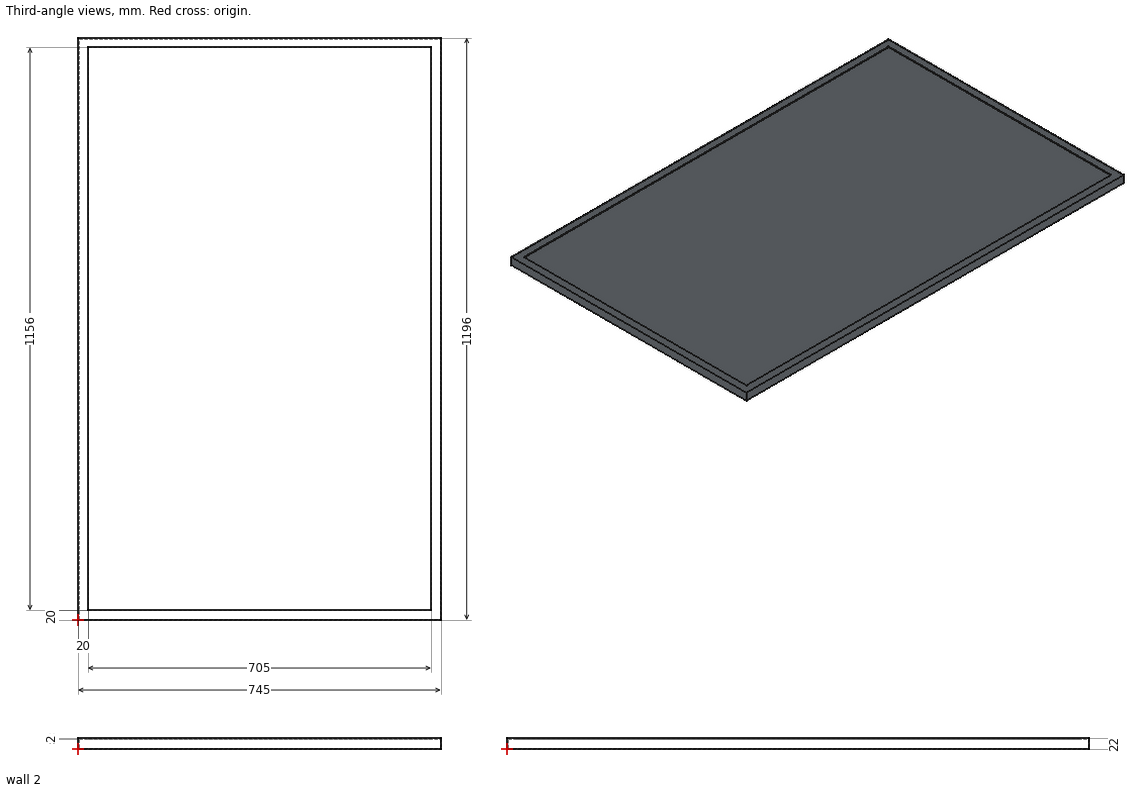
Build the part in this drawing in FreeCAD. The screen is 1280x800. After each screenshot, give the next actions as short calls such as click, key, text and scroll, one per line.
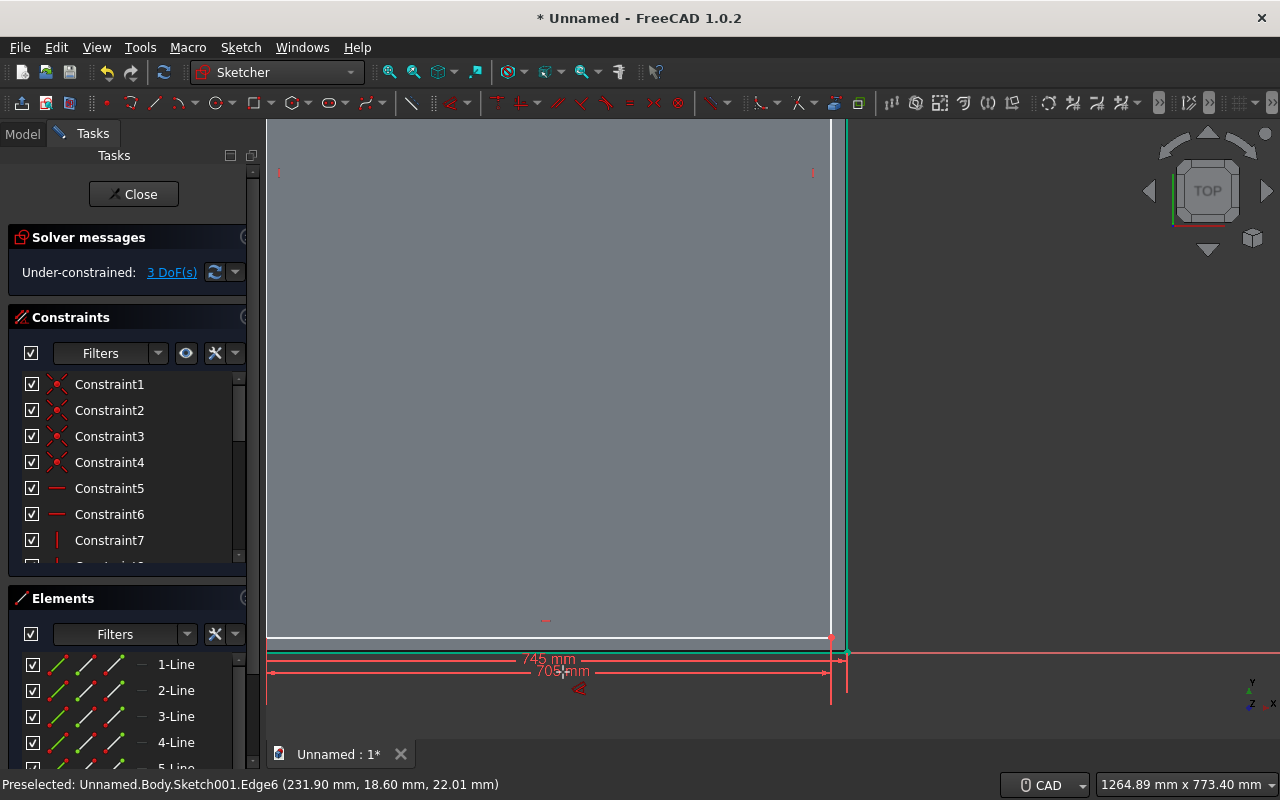
scroll(832, 637, down, 4)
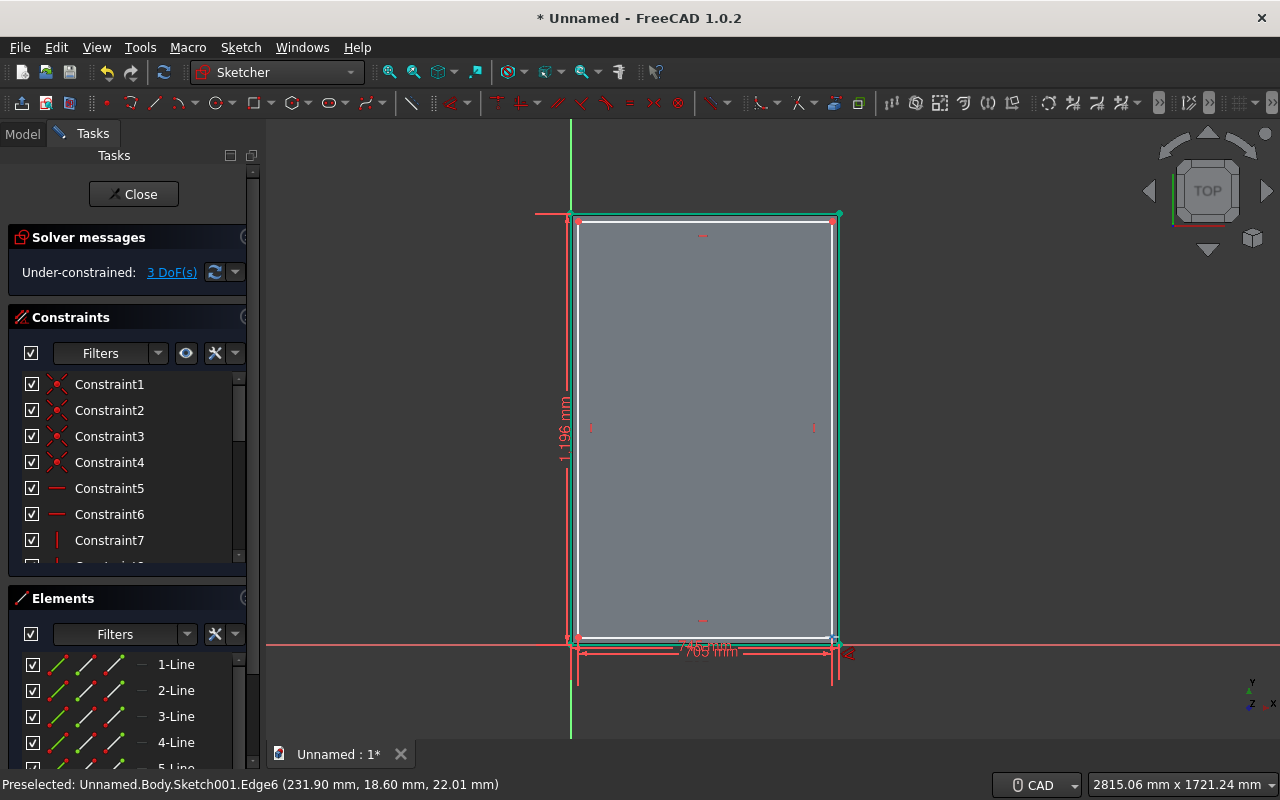
scroll(578, 222, up, 9)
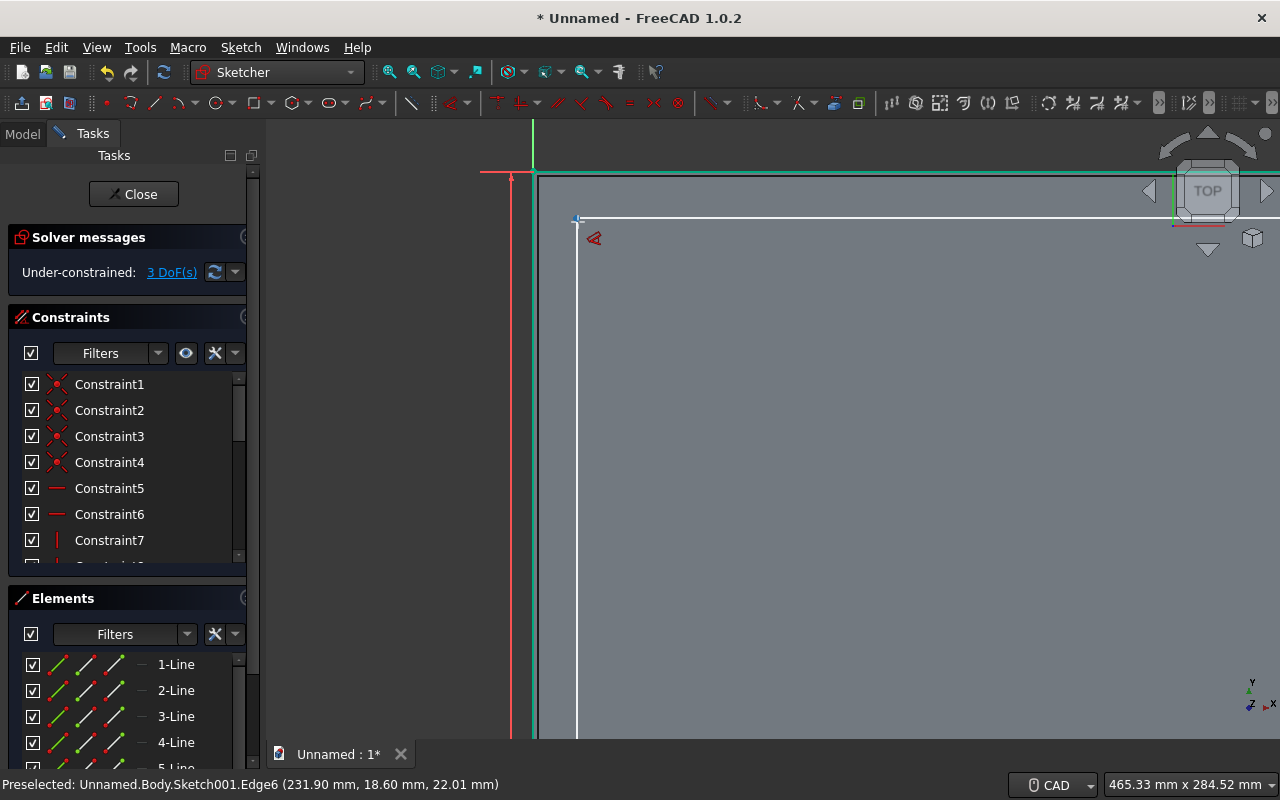
click(577, 218)
click(555, 184)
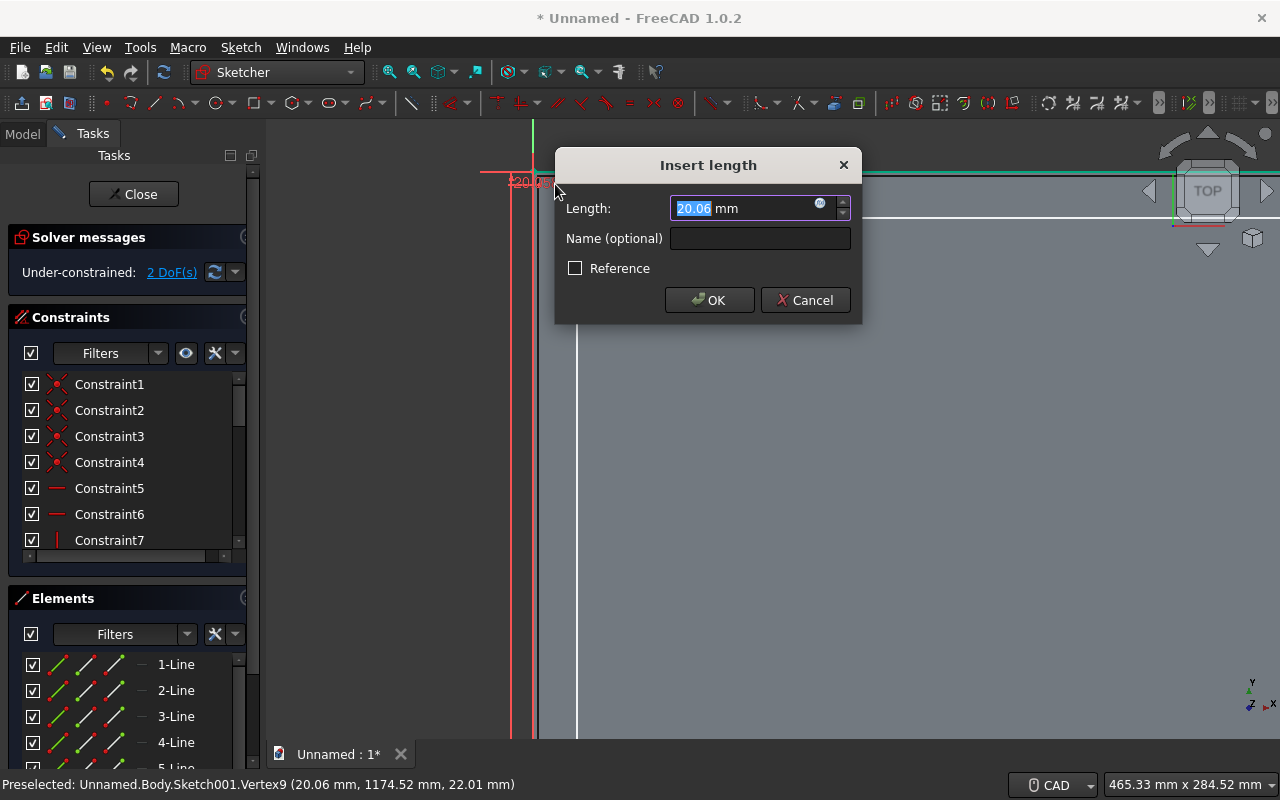
text(20)
key(Return)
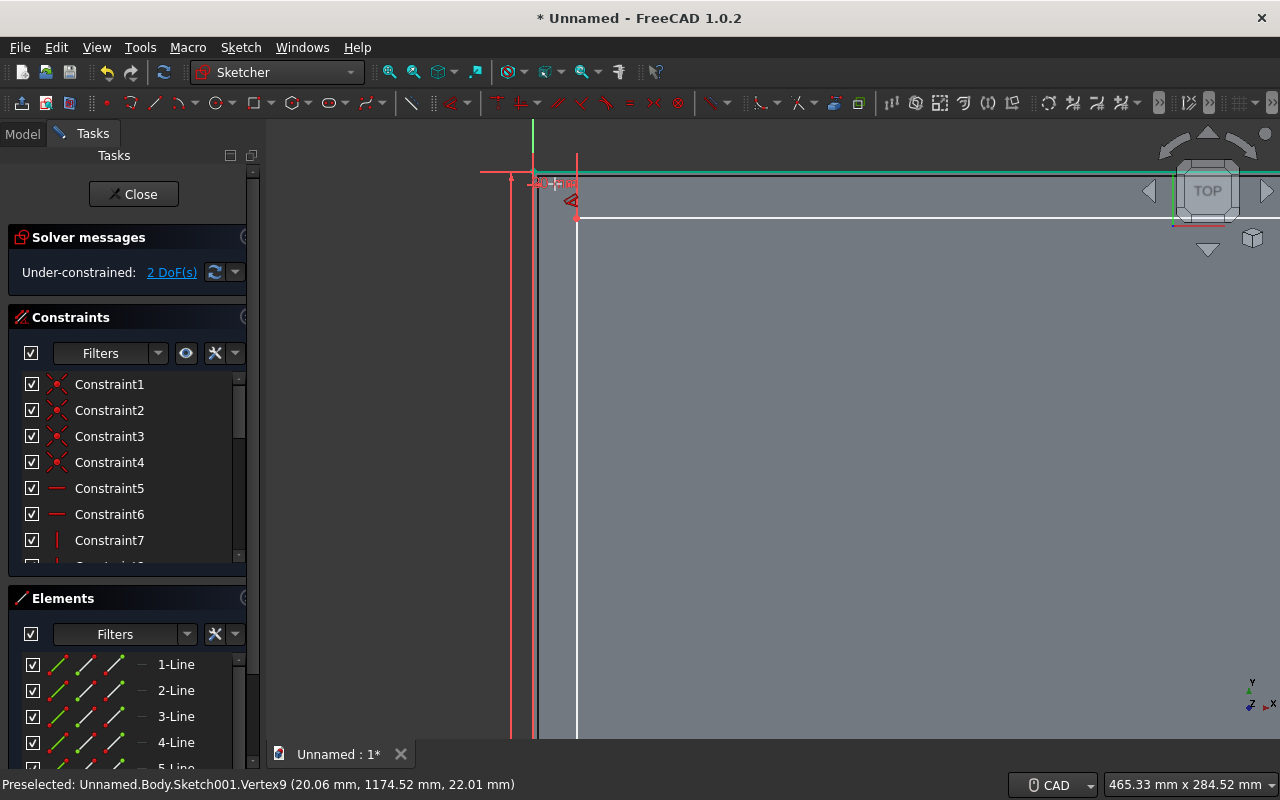
scroll(578, 222, down, 9)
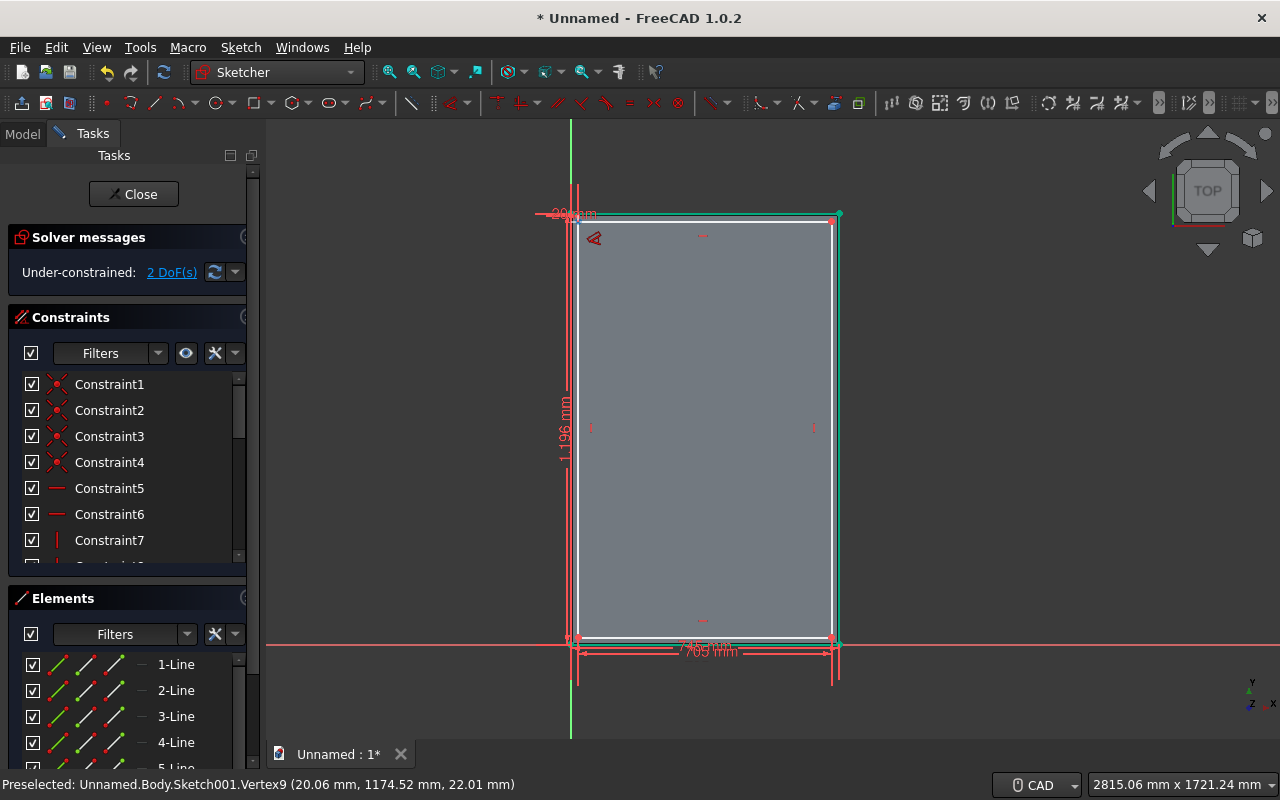
scroll(578, 638, up, 9)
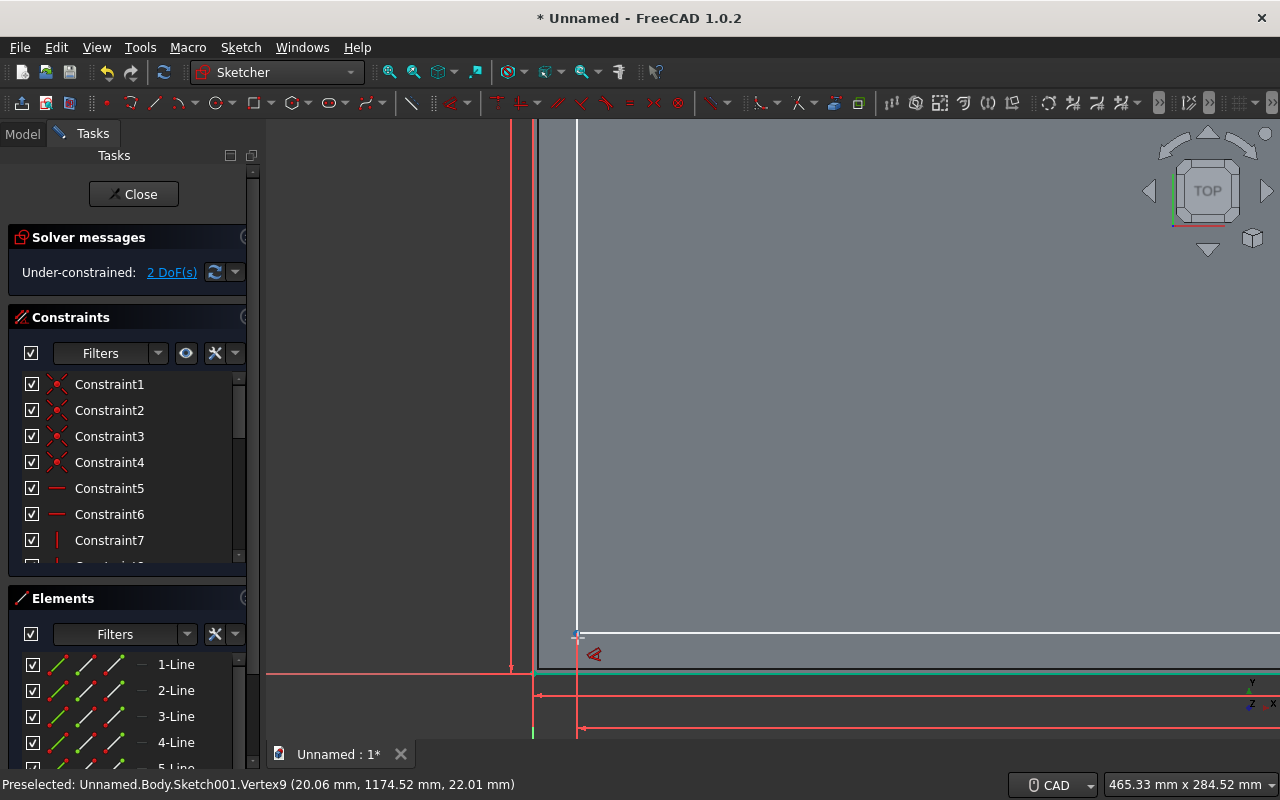
click(577, 633)
click(499, 653)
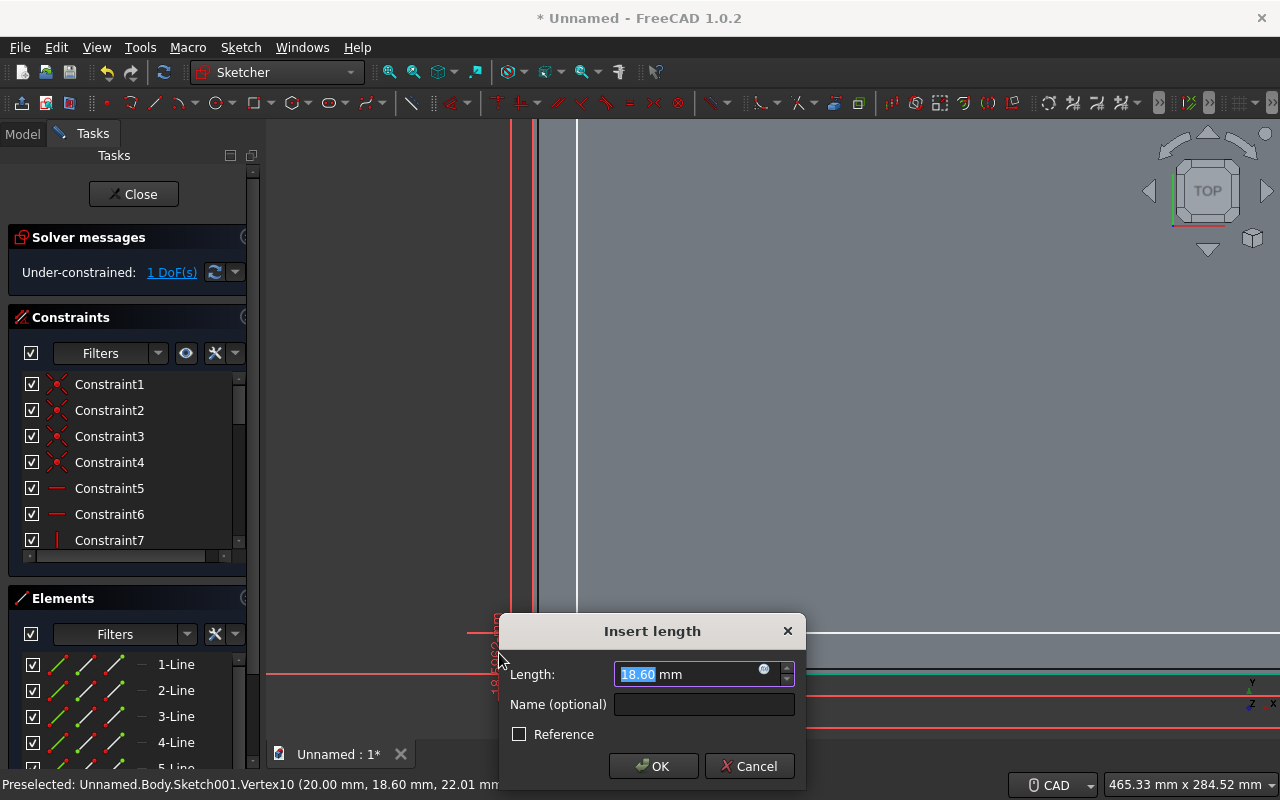
text(20)
key(Return)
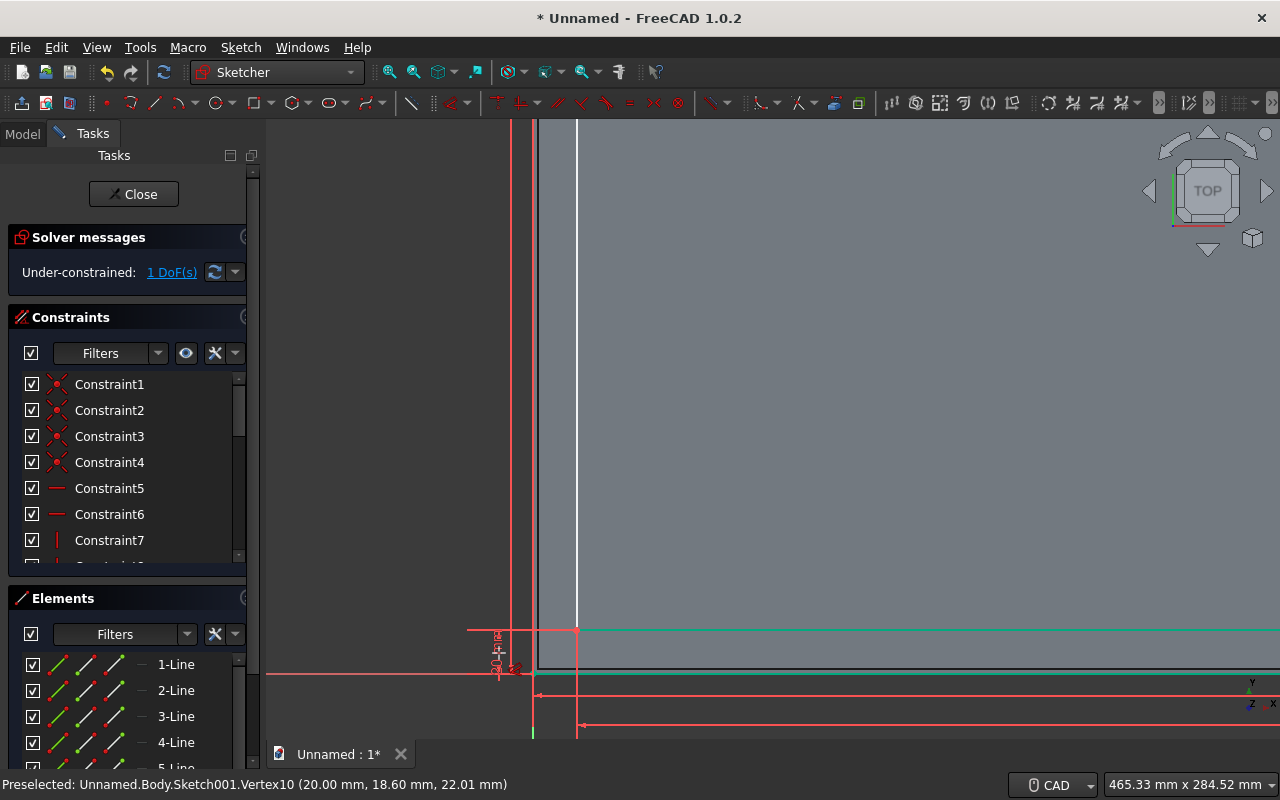
scroll(578, 639, down, 9)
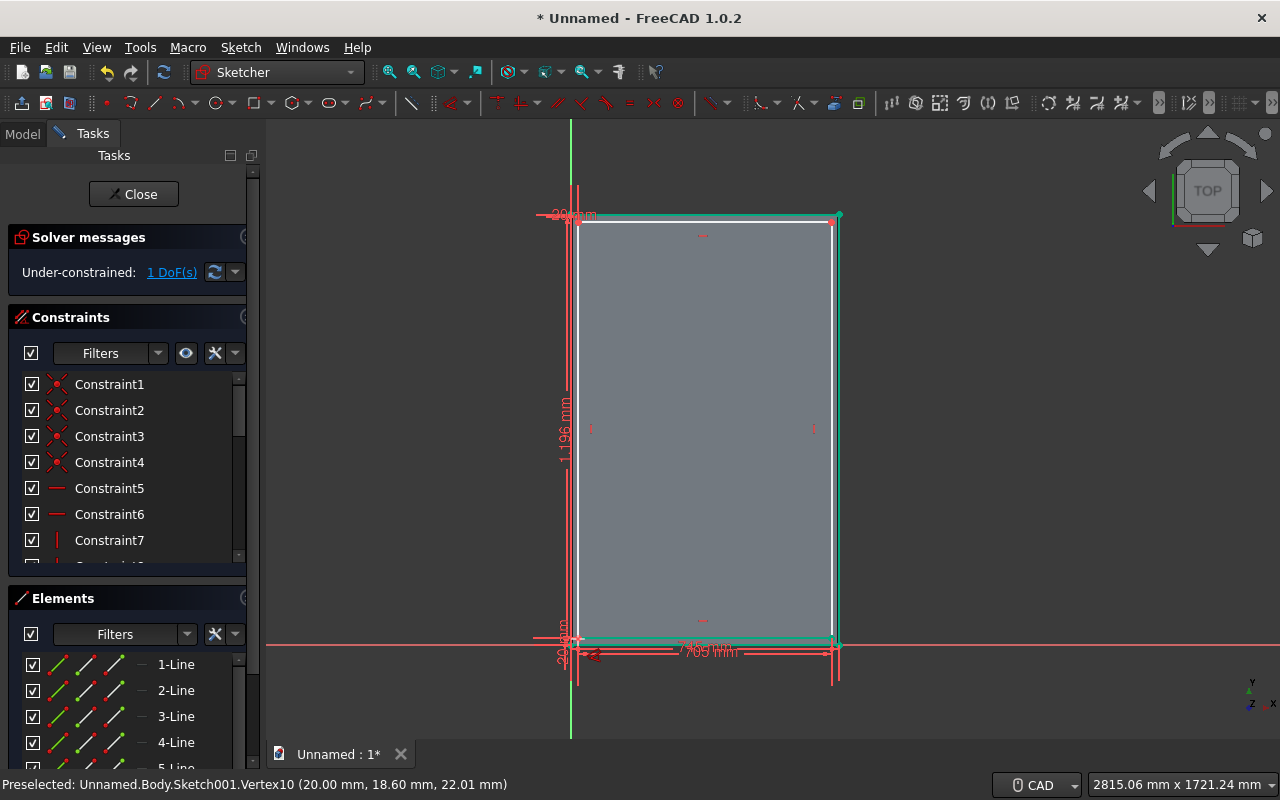
scroll(578, 347, up, 4)